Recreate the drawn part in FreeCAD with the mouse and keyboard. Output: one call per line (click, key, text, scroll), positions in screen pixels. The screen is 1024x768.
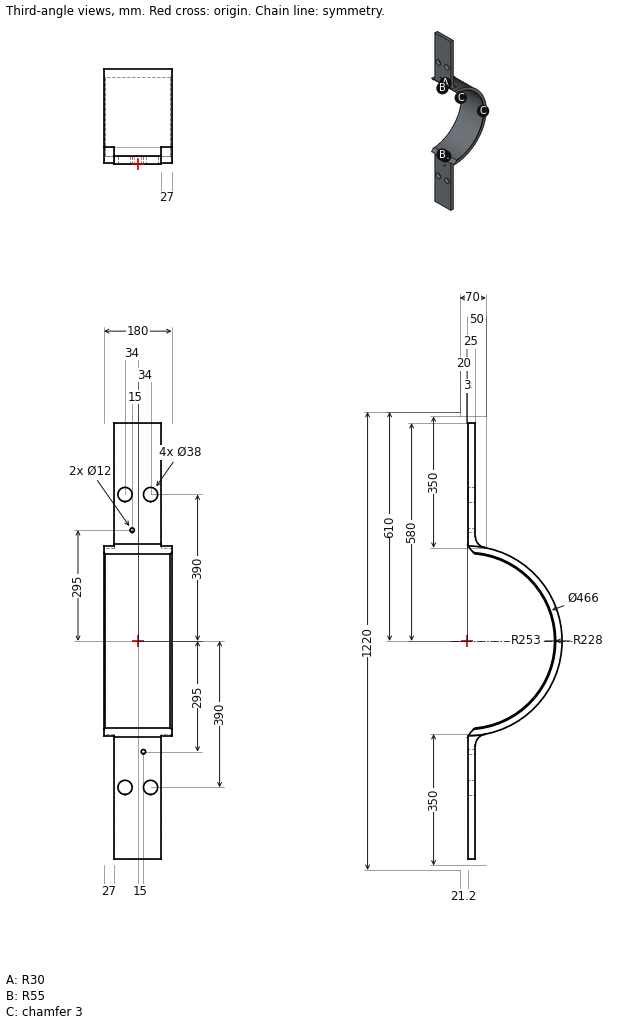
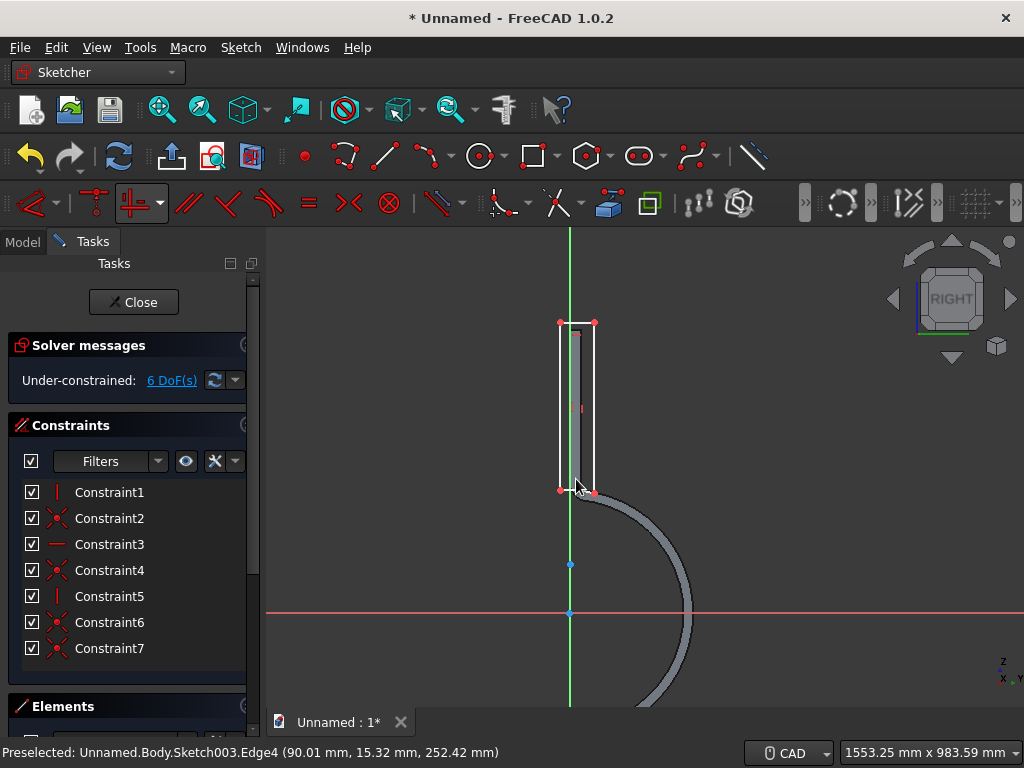
drag(560, 554, 581, 623)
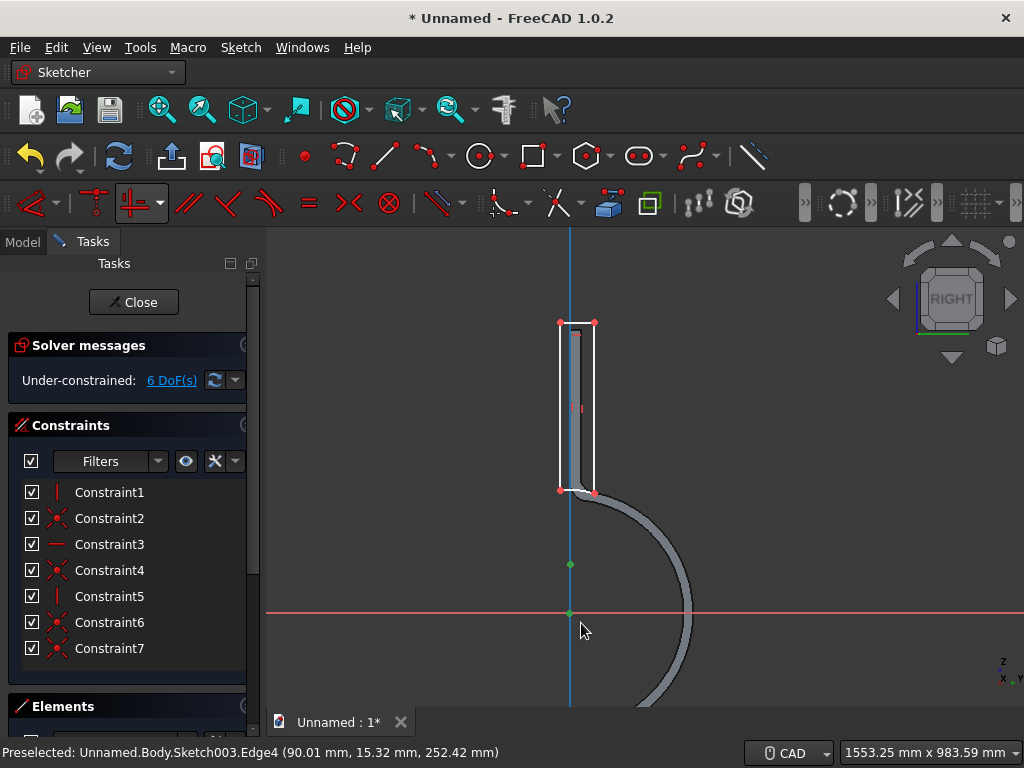
click(94, 204)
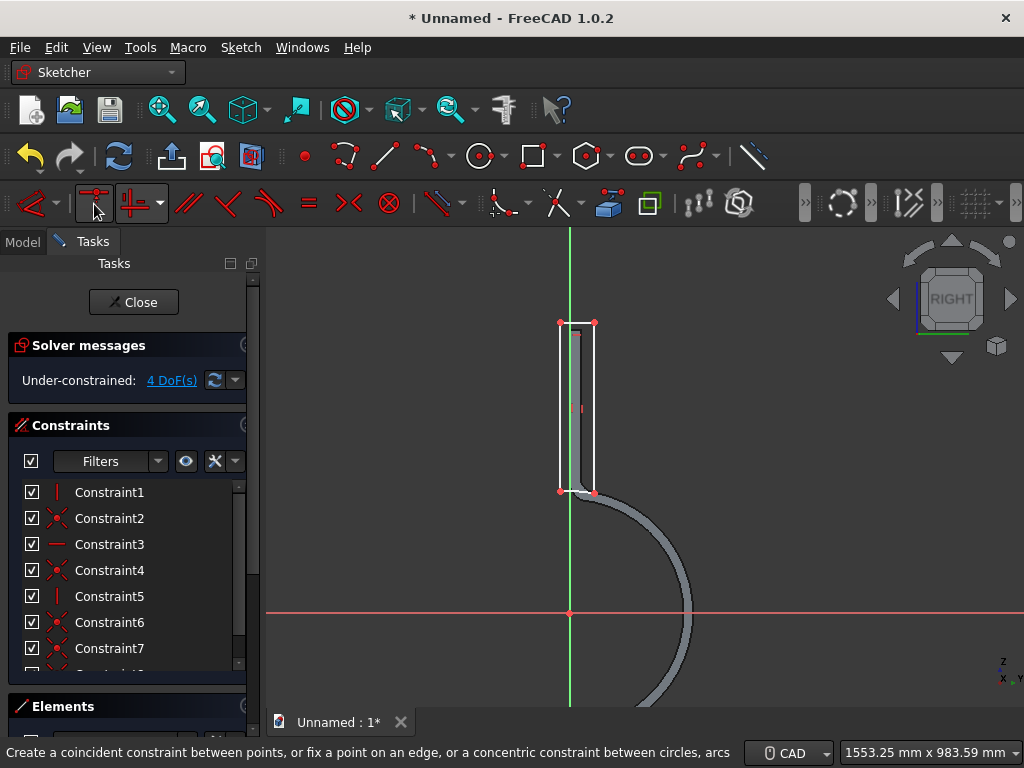
click(32, 204)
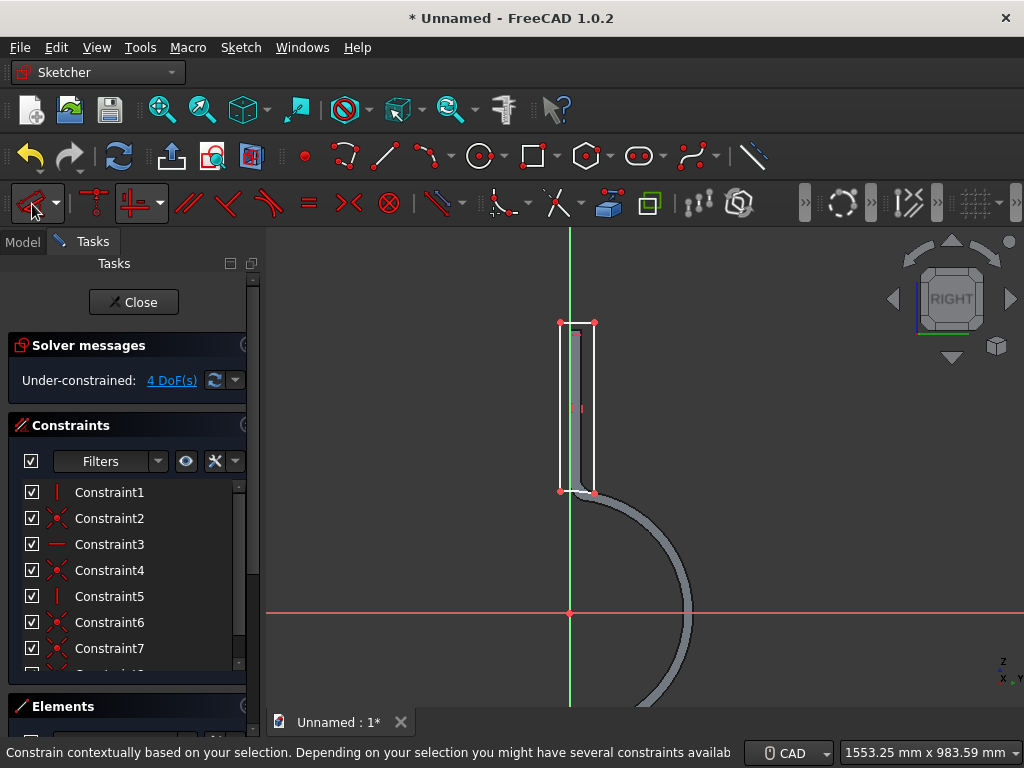
scroll(584, 492, up, 2)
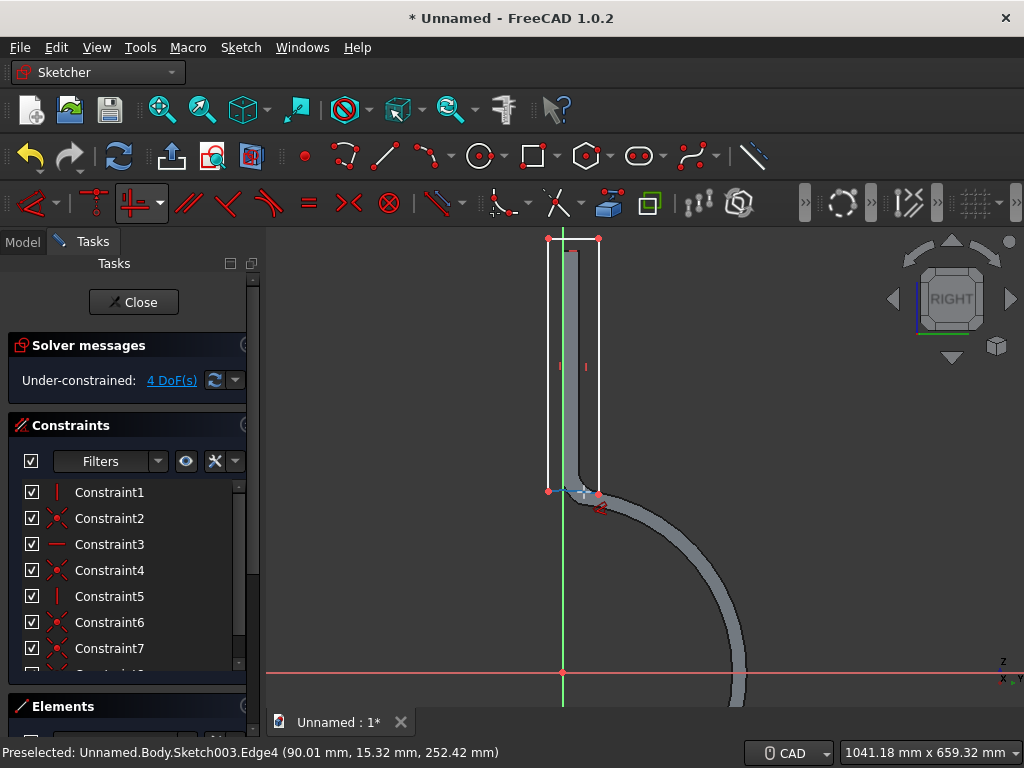
click(584, 492)
click(687, 498)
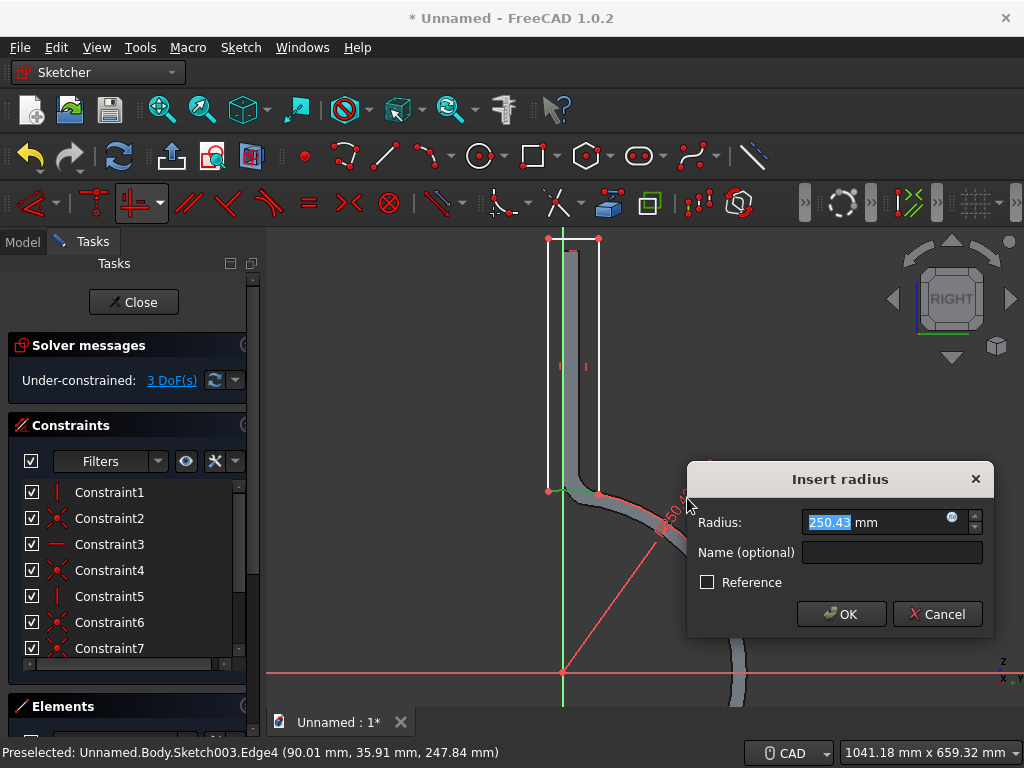
text(253)
key(Return)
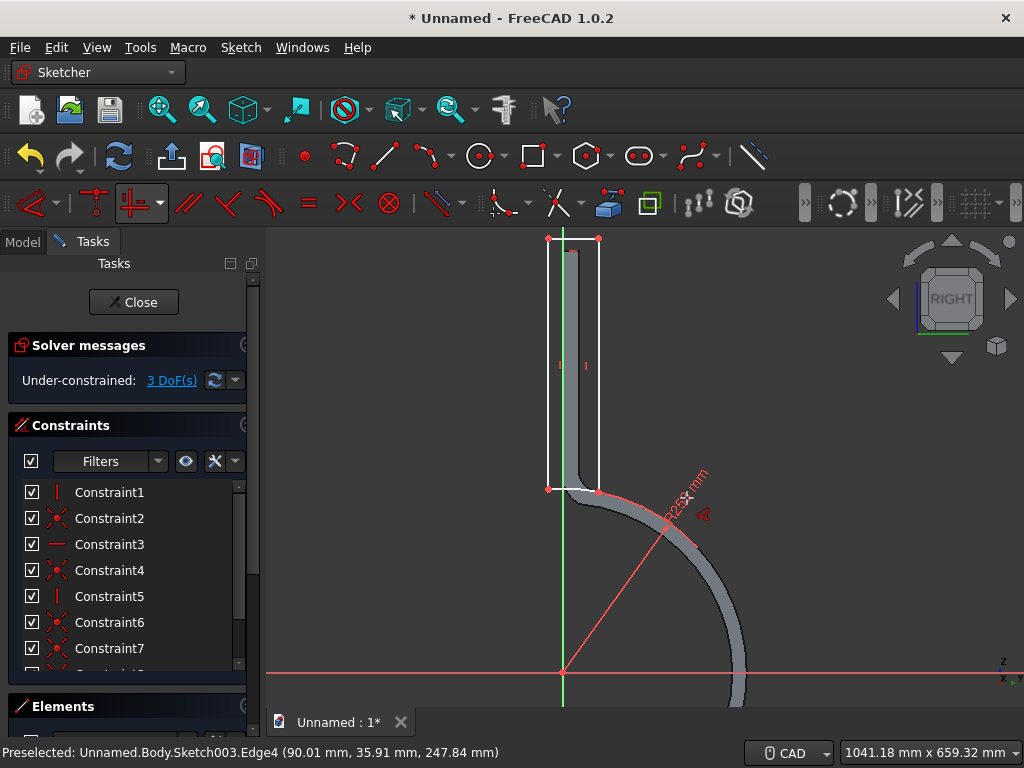
scroll(583, 491, down, 2)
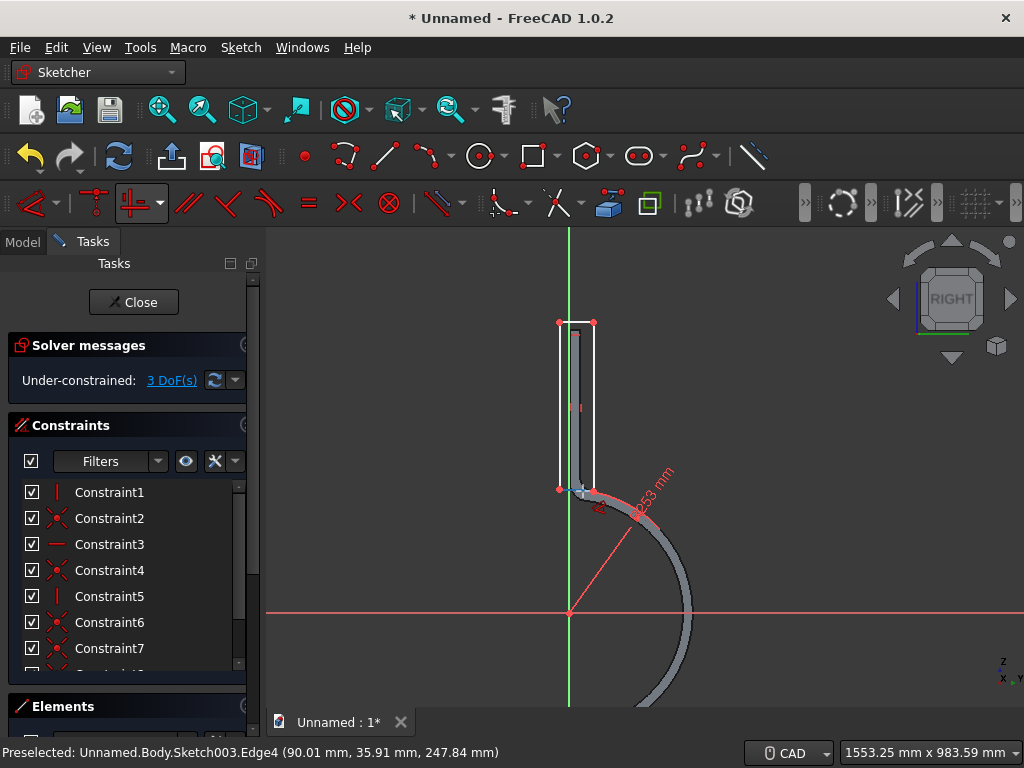
scroll(584, 322, up, 2)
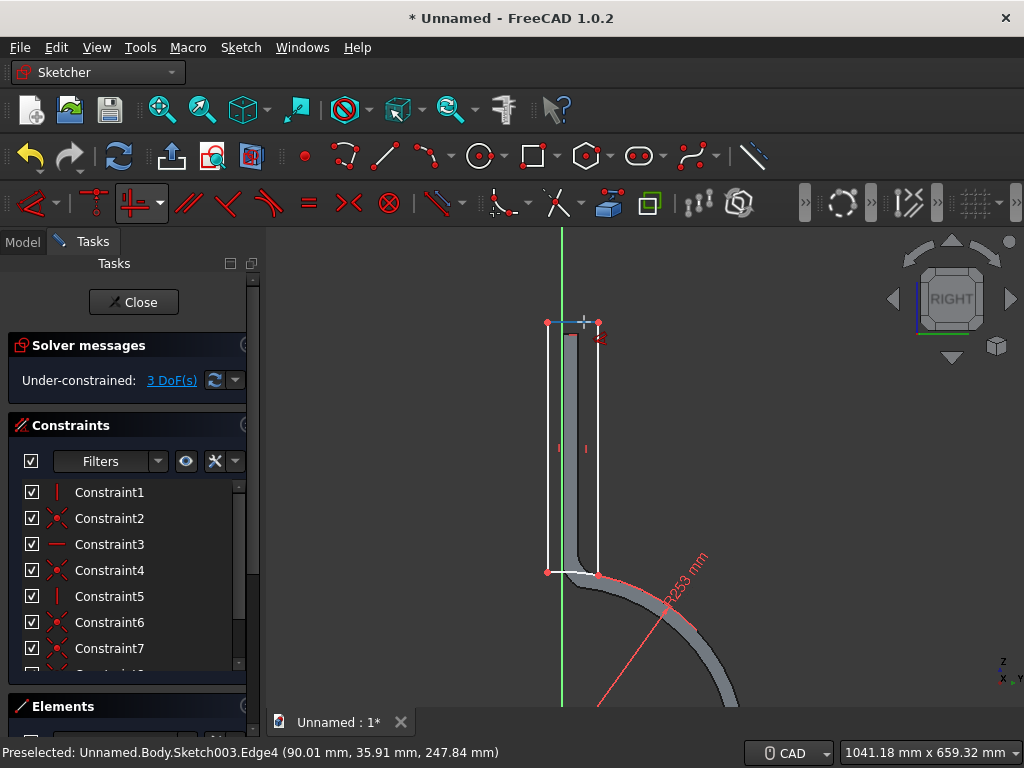
click(583, 322)
click(585, 288)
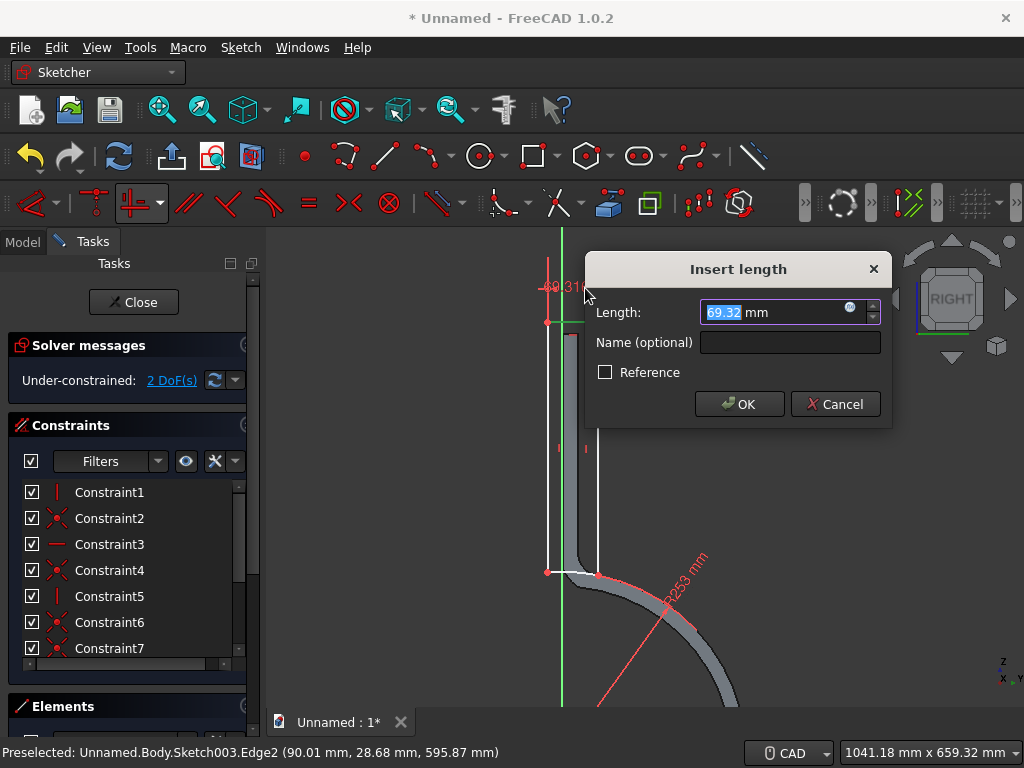
text(70)
key(Return)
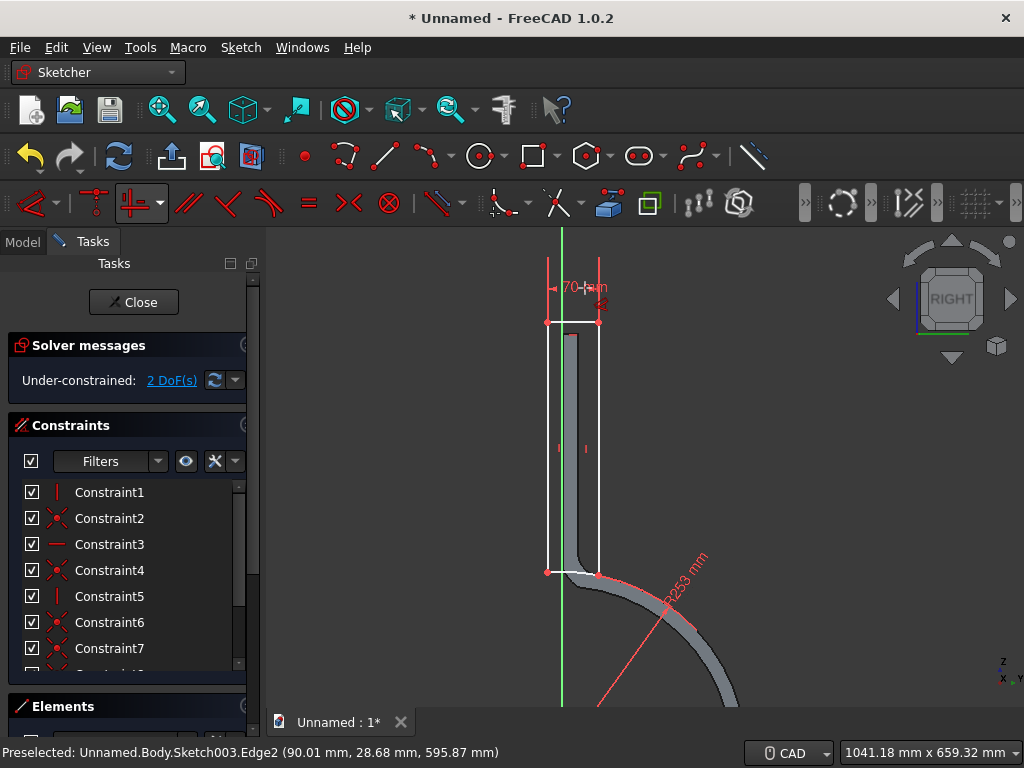
click(599, 500)
click(633, 449)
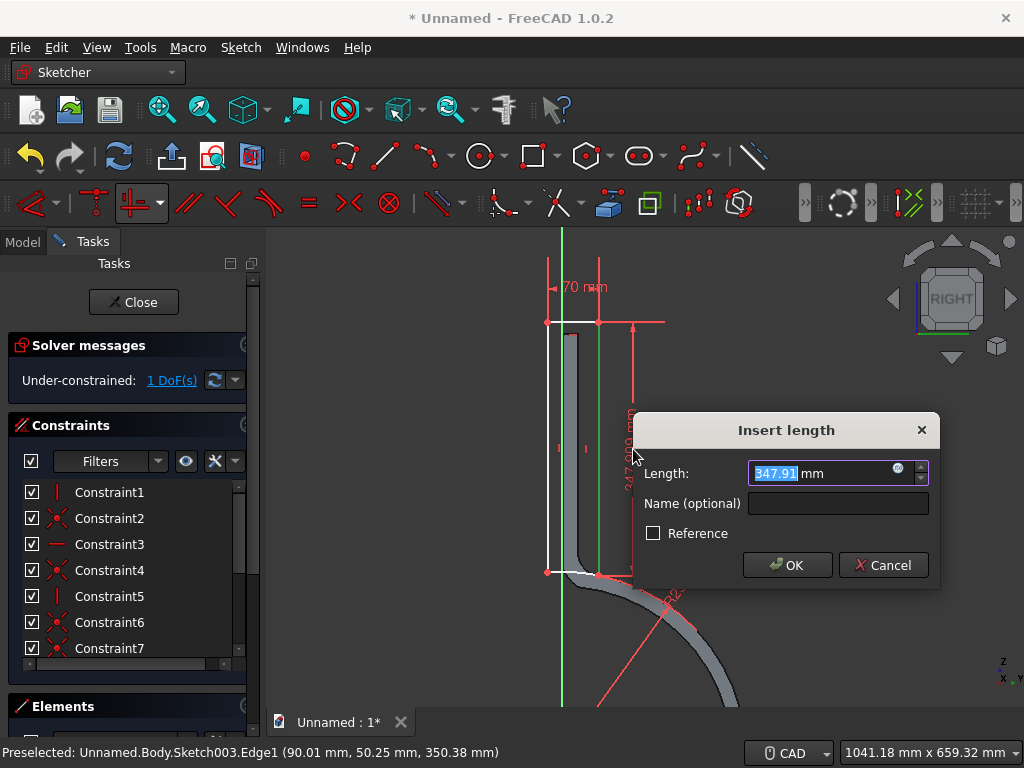
text(350)
key(Return)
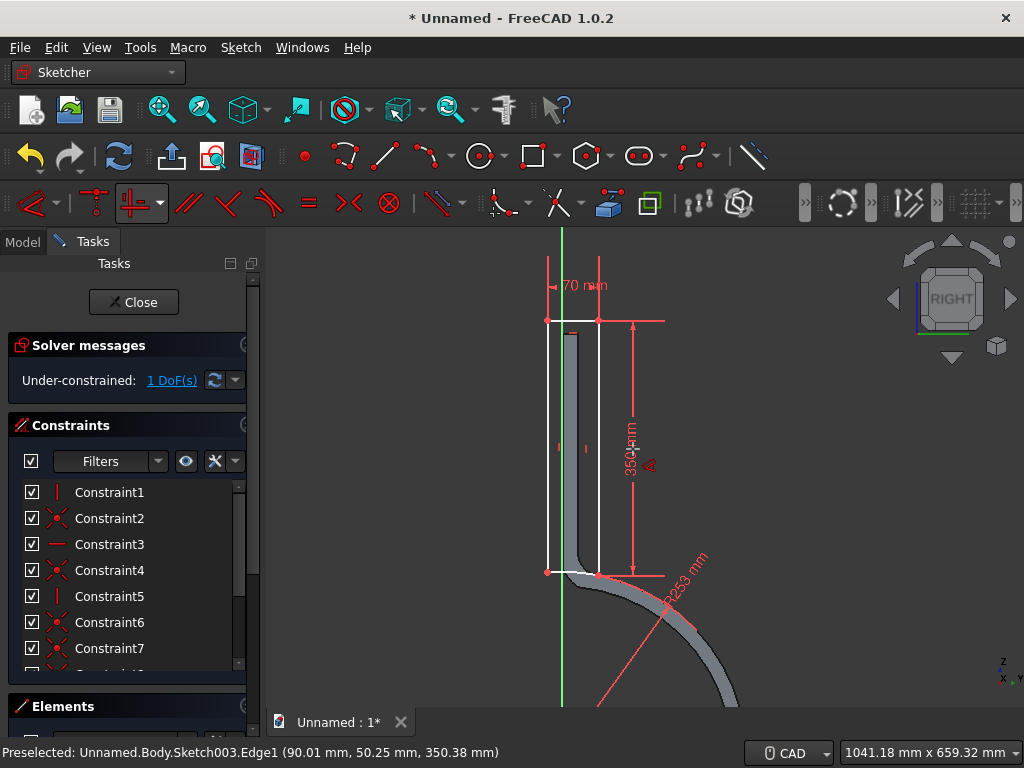
click(599, 576)
click(580, 542)